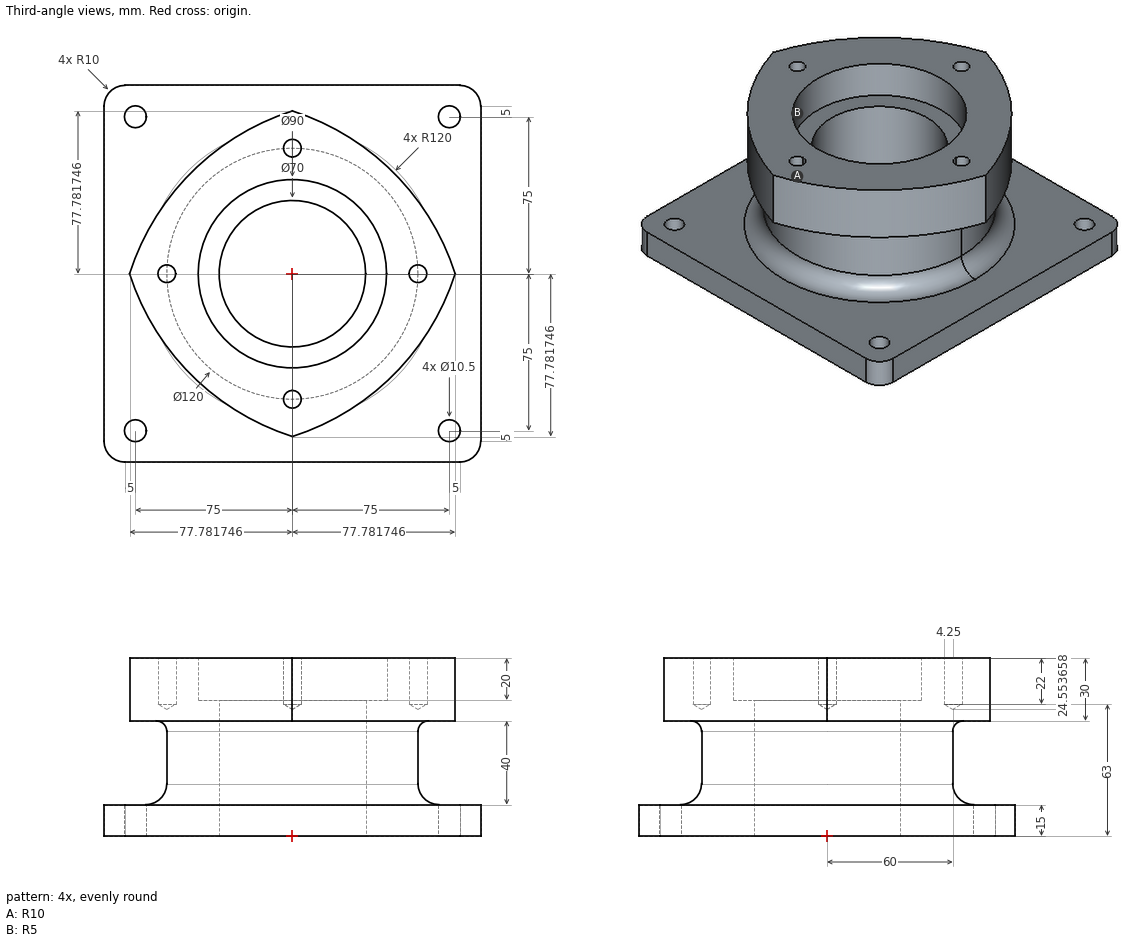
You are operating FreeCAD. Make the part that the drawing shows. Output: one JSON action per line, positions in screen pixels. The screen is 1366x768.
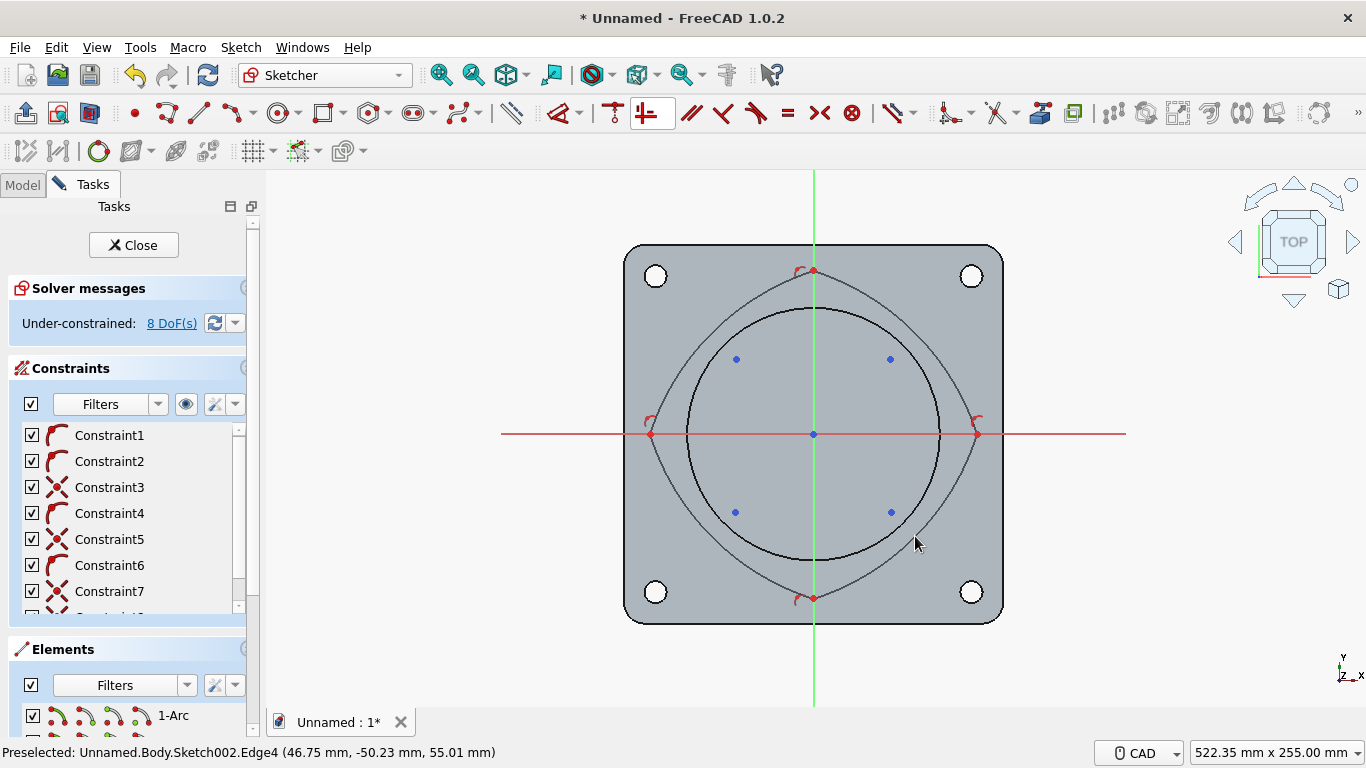
{"action": "left_click", "coordinate": [945, 370]}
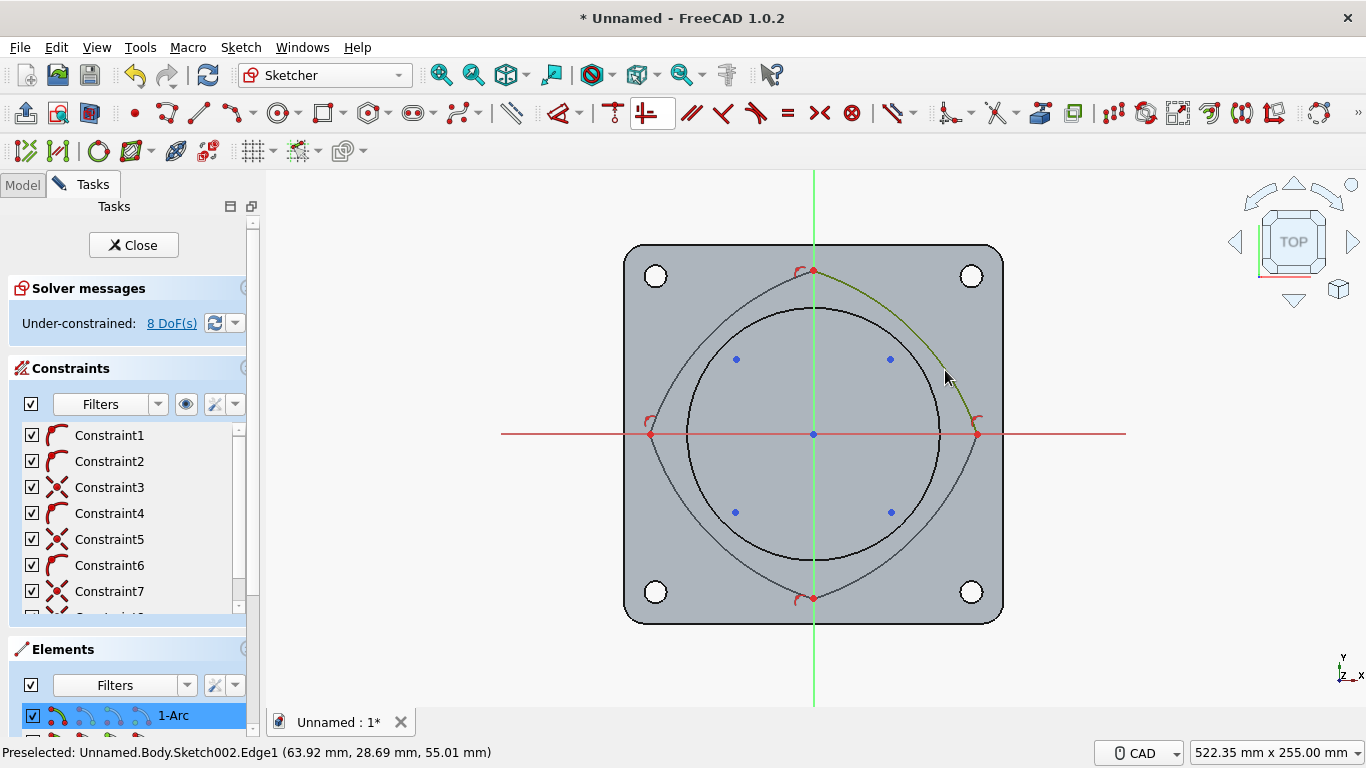
{"action": "left_click", "coordinate": [749, 302]}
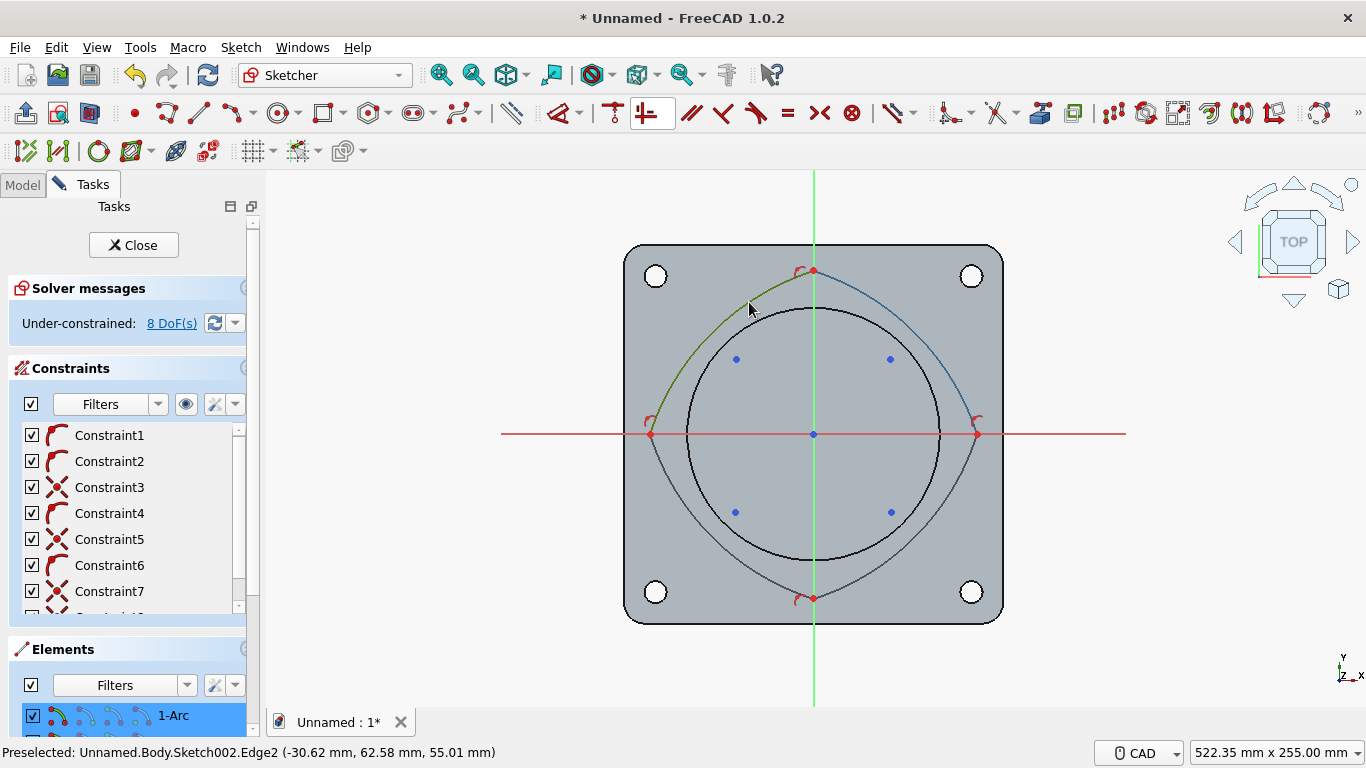
{"action": "left_click", "coordinate": [681, 499]}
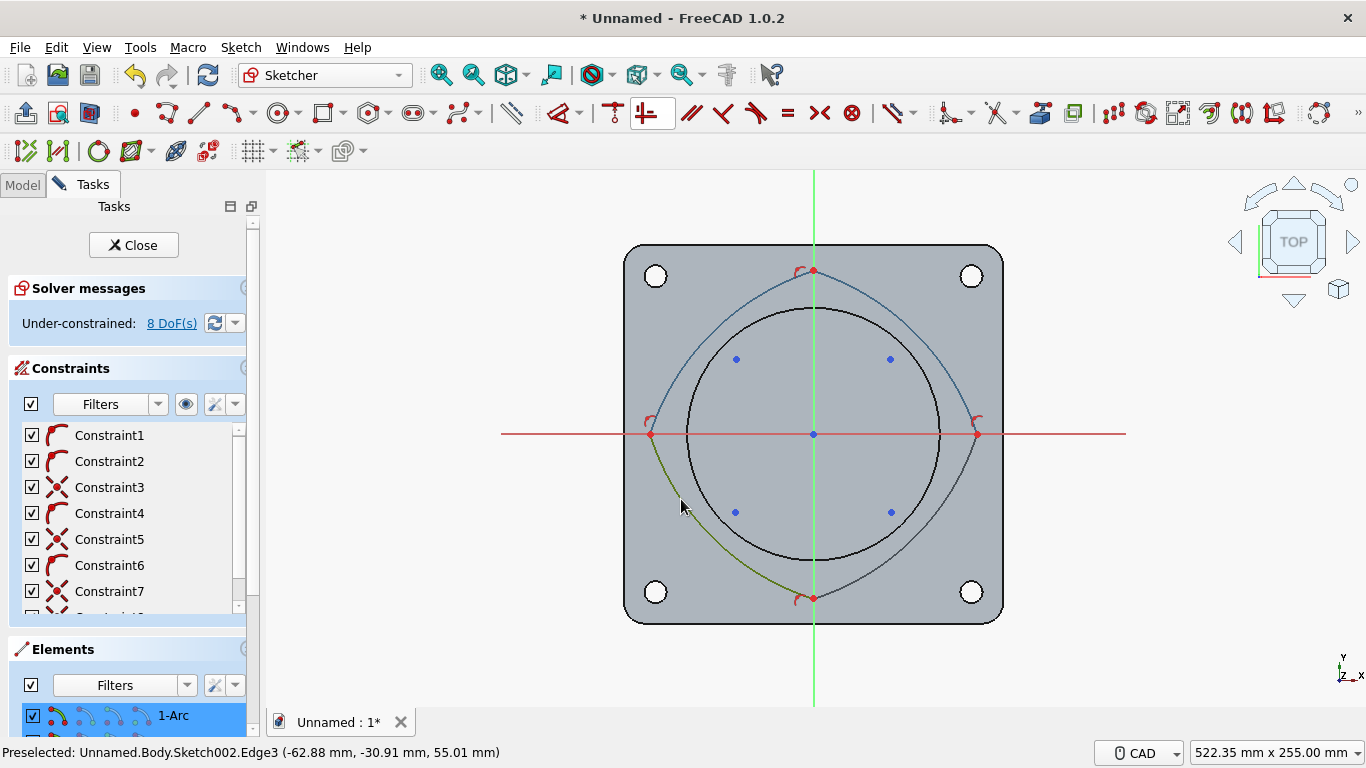
{"action": "left_click", "coordinate": [878, 567]}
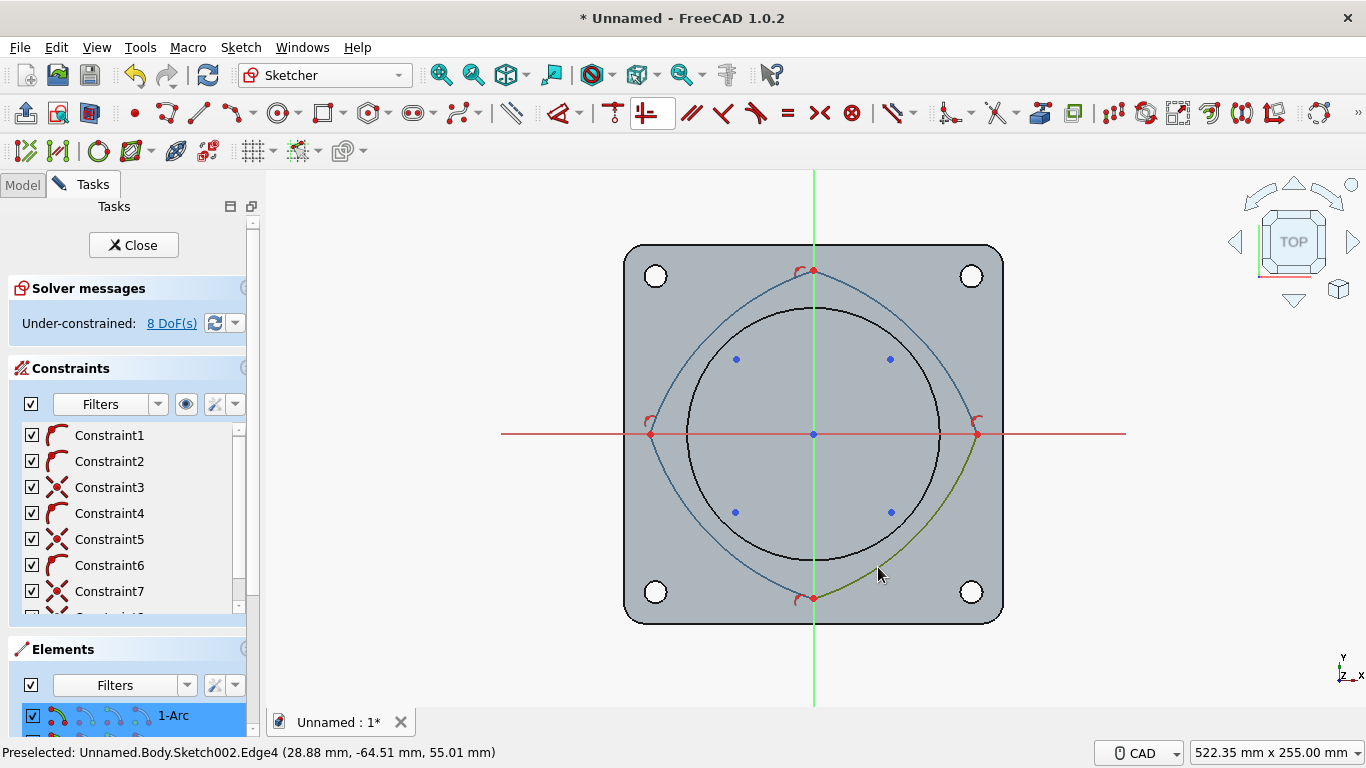
{"action": "left_click", "coordinate": [788, 114]}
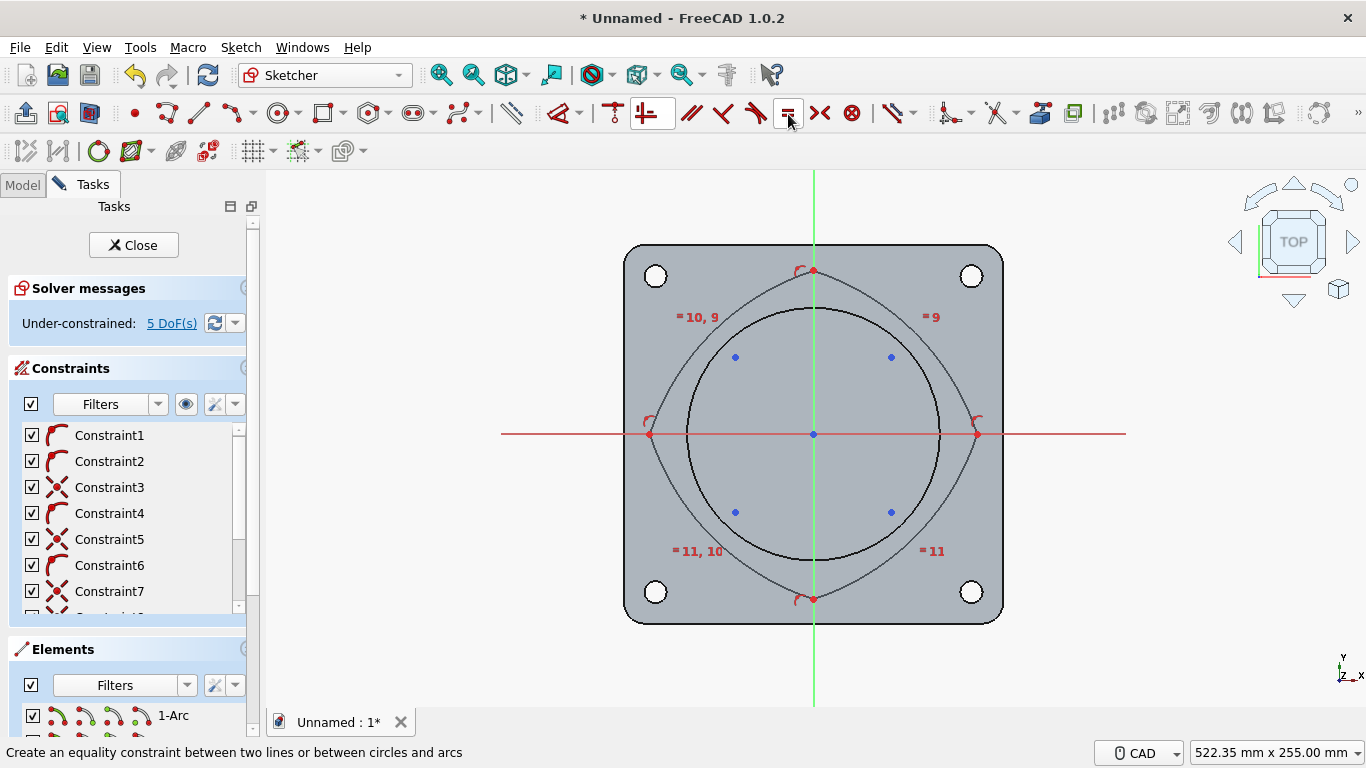
{"action": "left_click", "coordinate": [558, 114]}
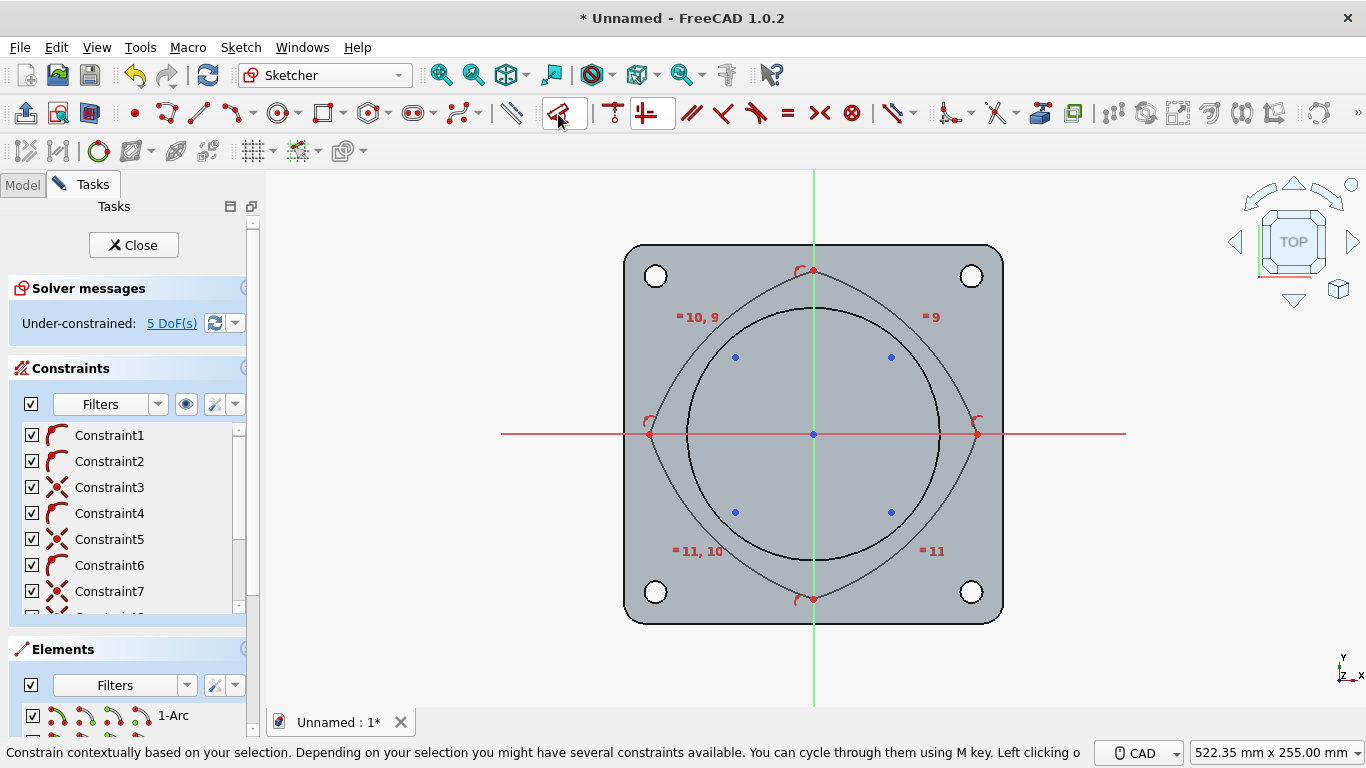
{"action": "left_click", "coordinate": [946, 370]}
{"action": "left_click", "coordinate": [972, 352]}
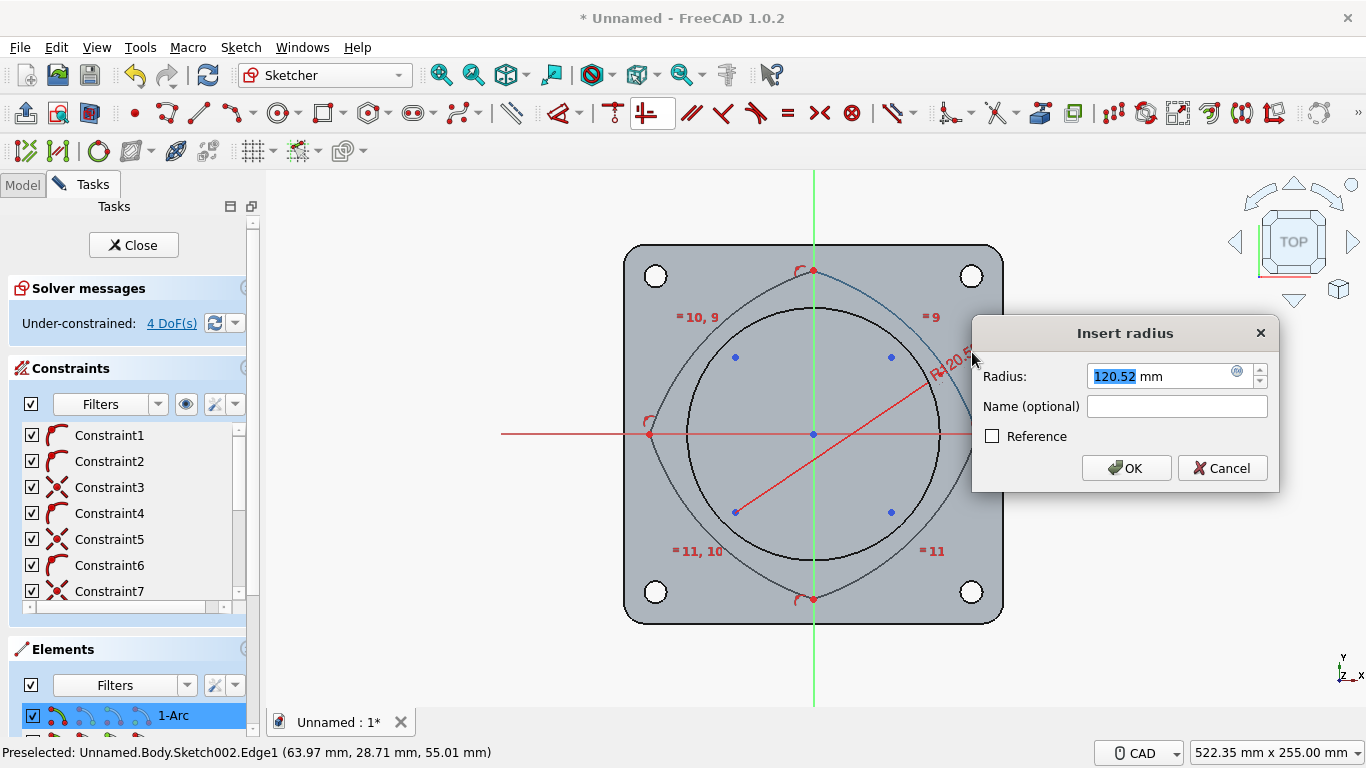
{"action": "type", "text": "120"}
{"action": "key", "text": "Return"}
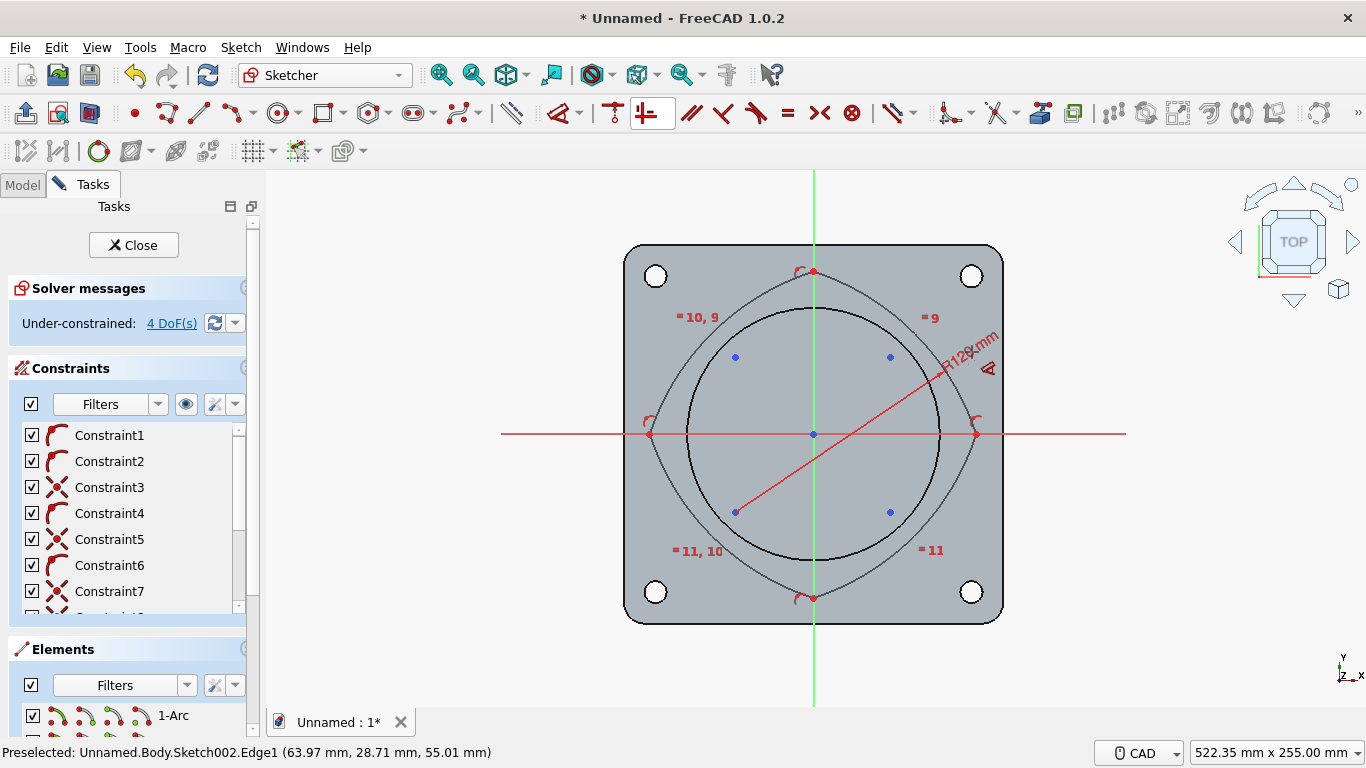
{"action": "left_click", "coordinate": [976, 434]}
{"action": "left_click", "coordinate": [895, 468]}